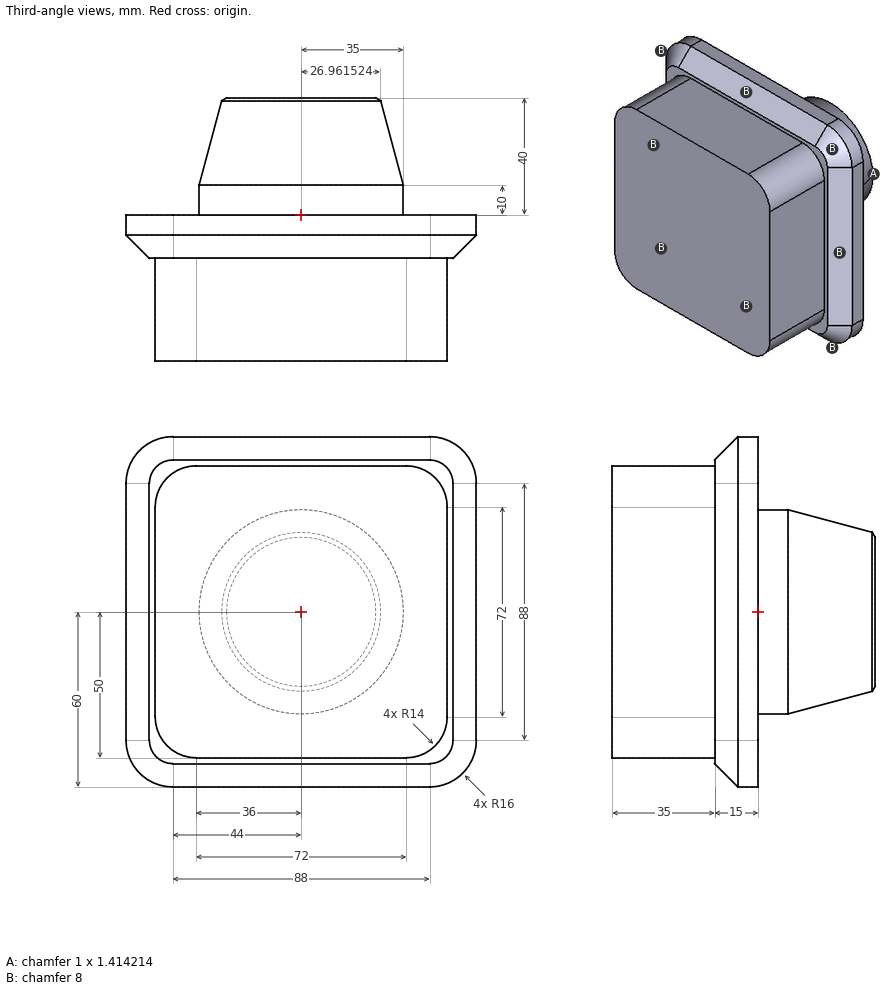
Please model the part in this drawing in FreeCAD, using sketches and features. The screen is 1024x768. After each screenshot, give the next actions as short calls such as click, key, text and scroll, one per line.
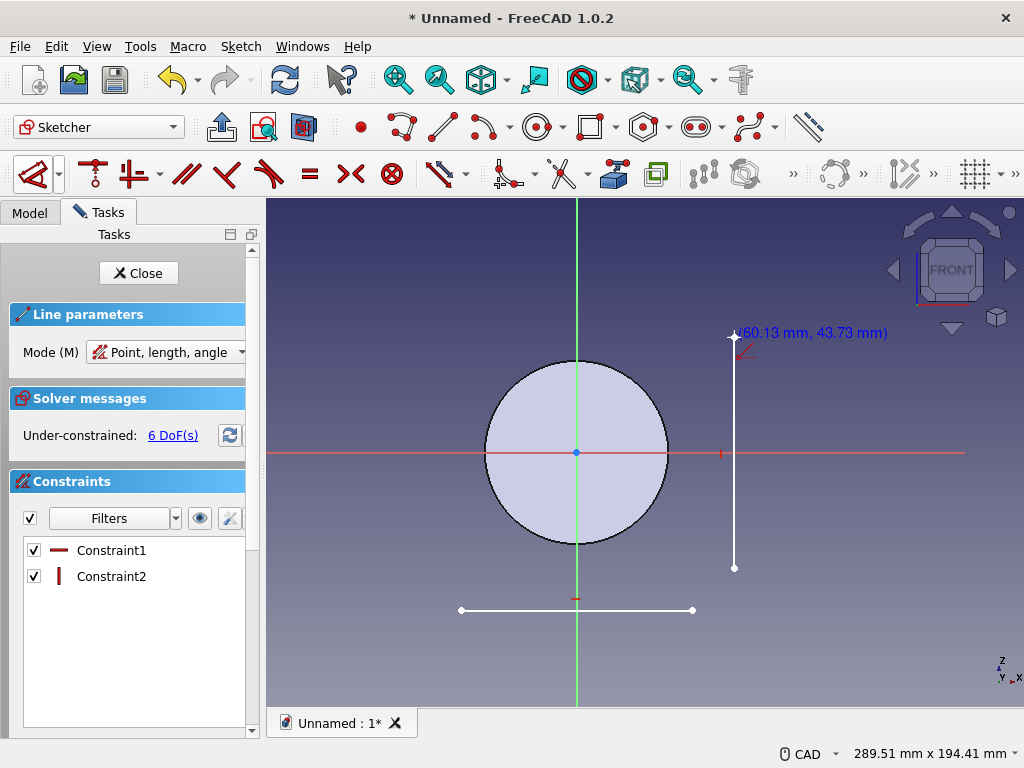
click(692, 295)
click(461, 295)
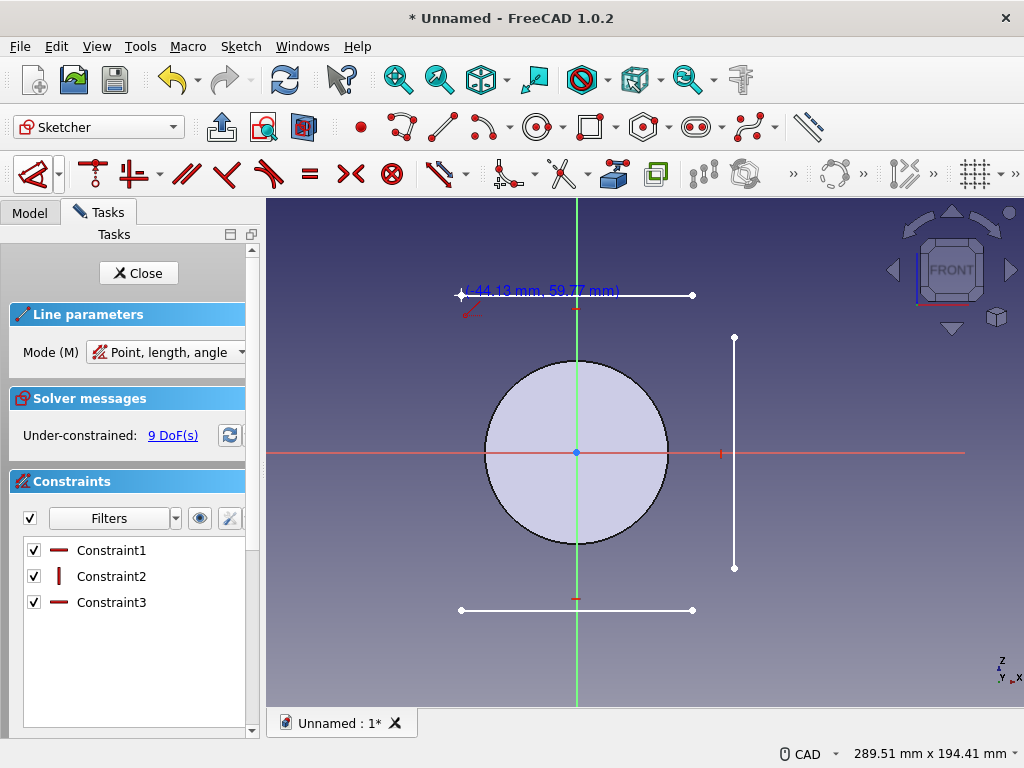
click(419, 337)
click(419, 568)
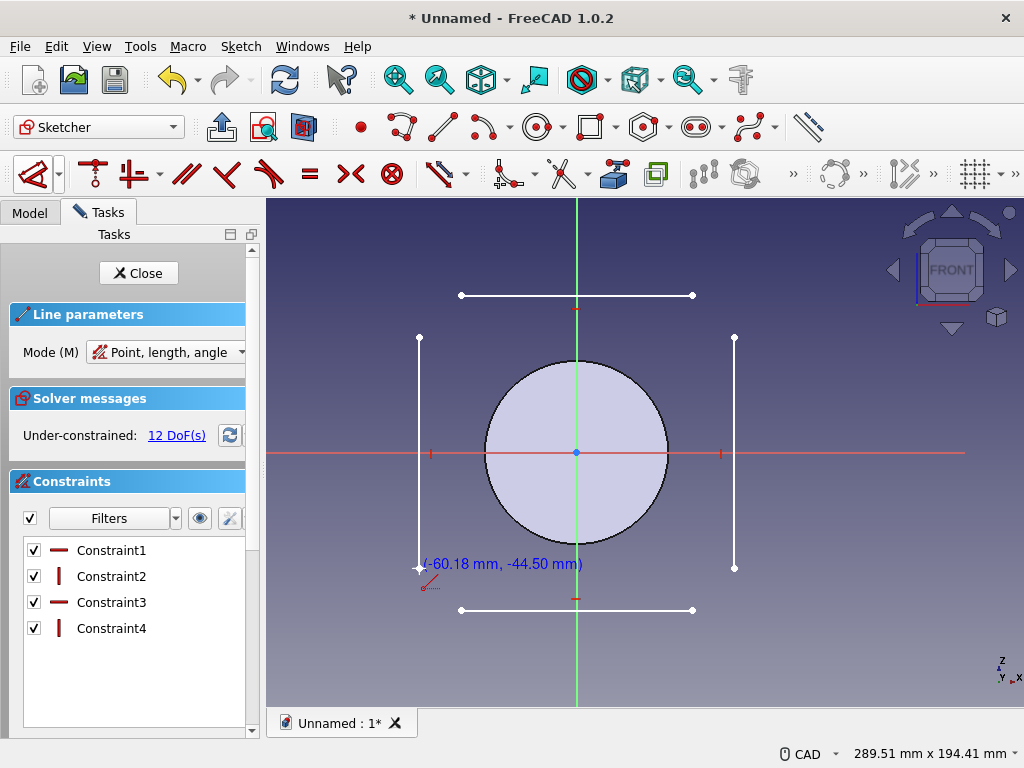
key(g)
key(3)
key(a)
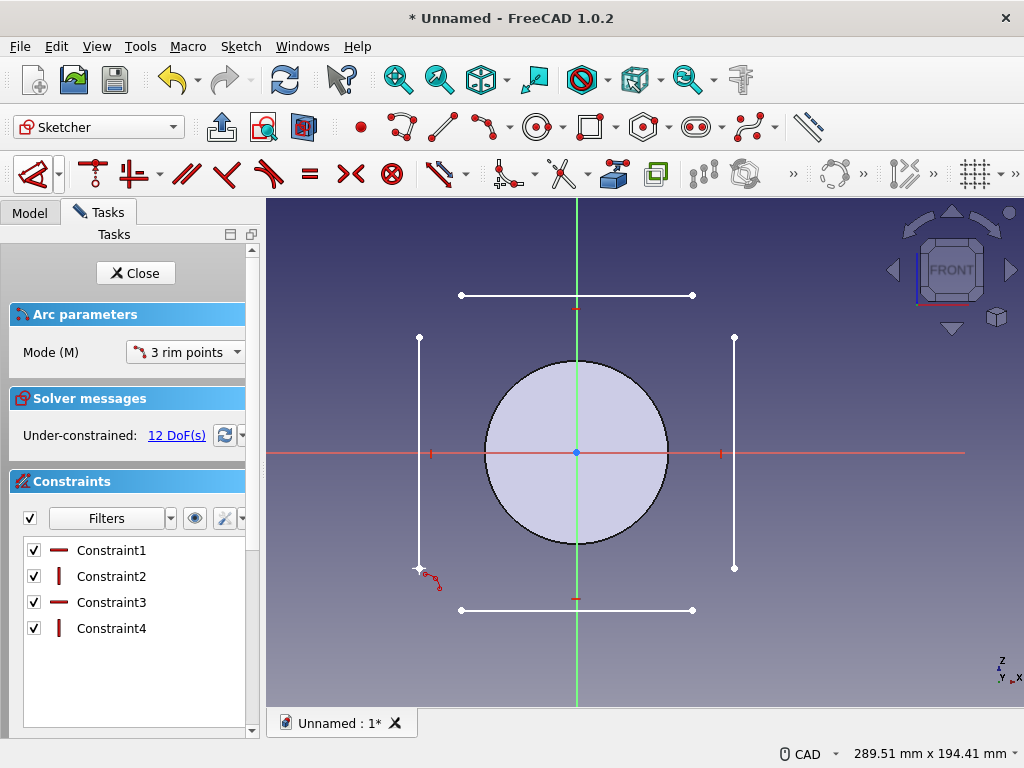
click(692, 611)
click(734, 569)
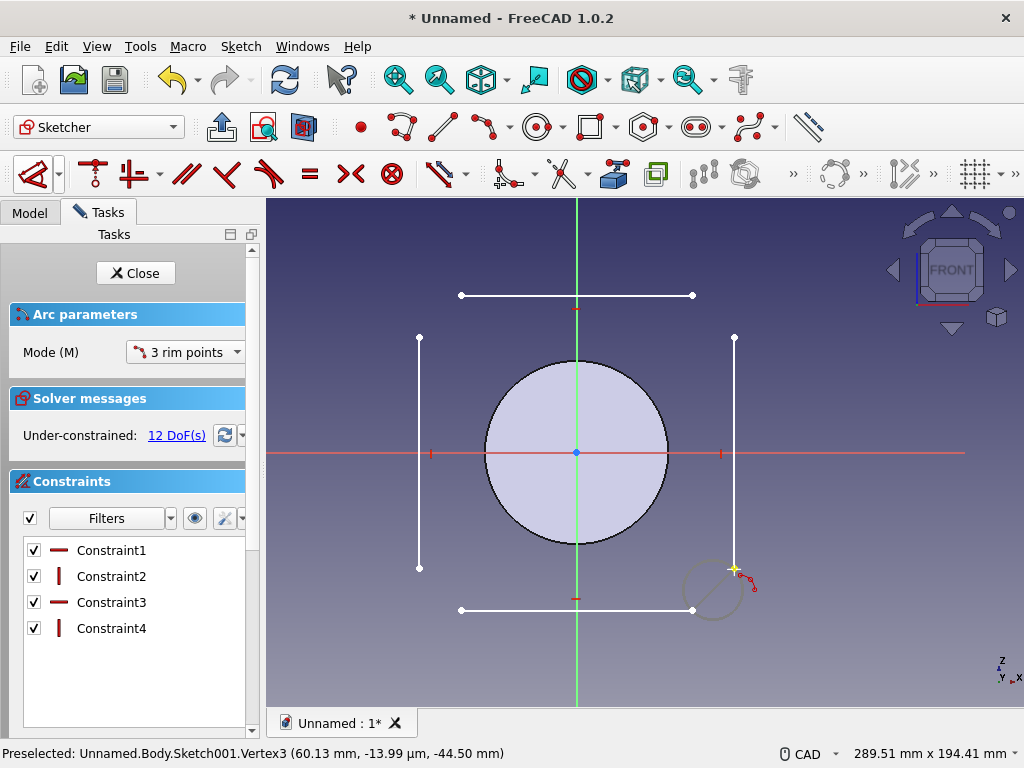
scroll(721, 597, up, 2)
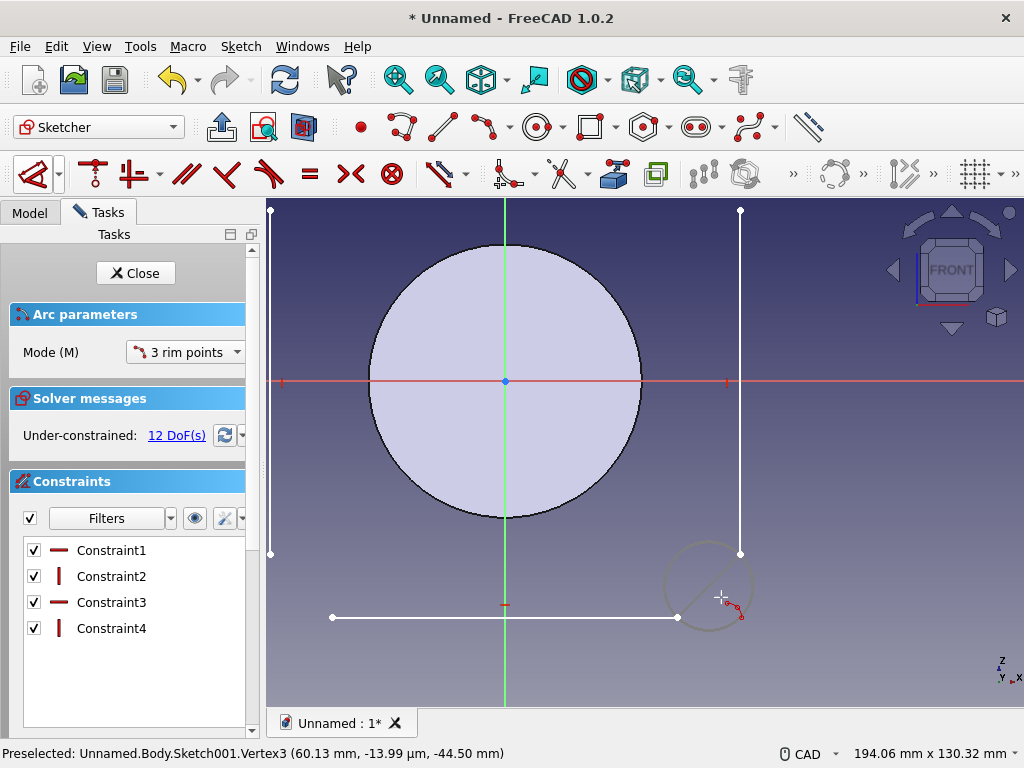
click(721, 597)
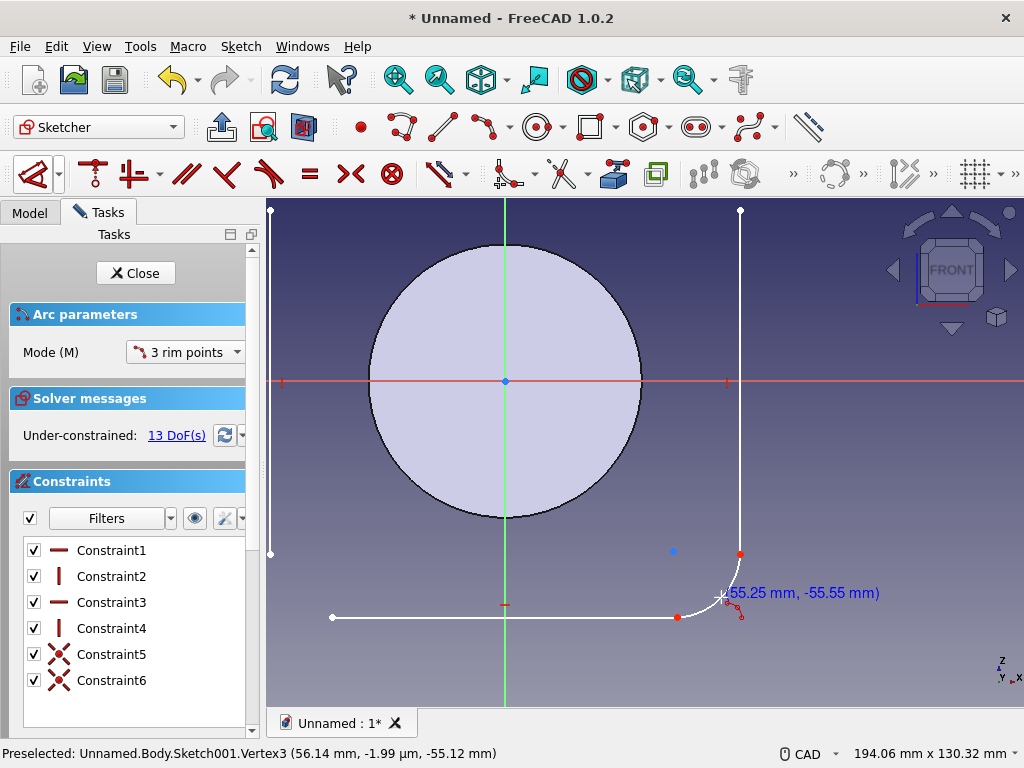
scroll(721, 598, down, 2)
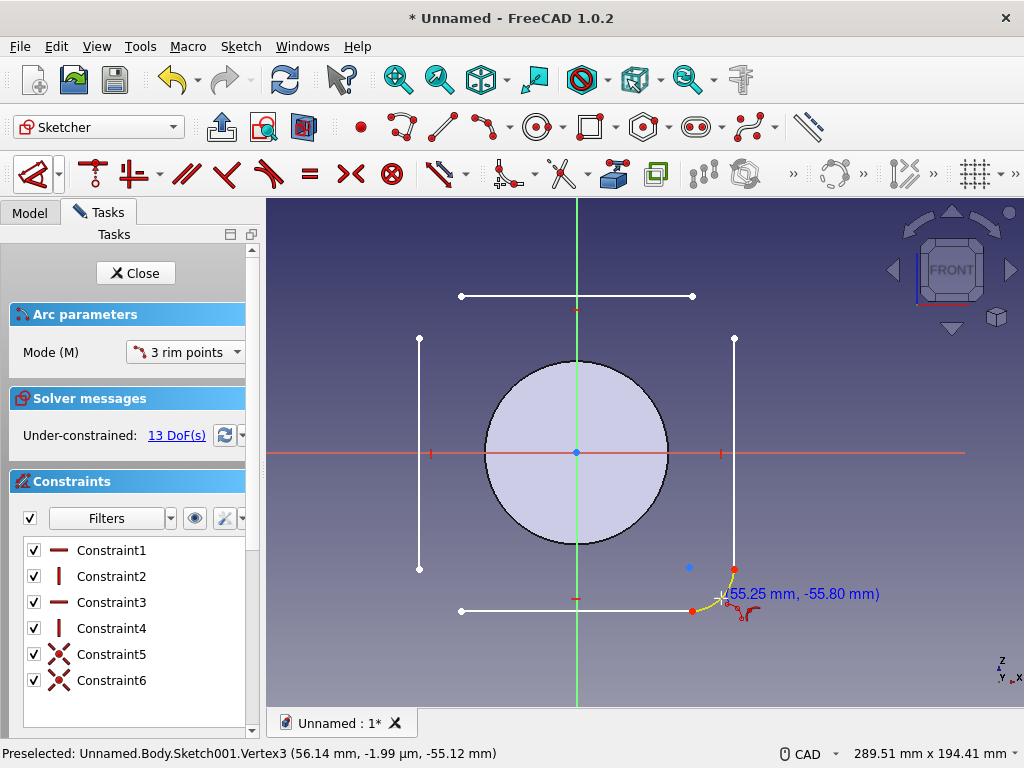
click(734, 338)
click(692, 296)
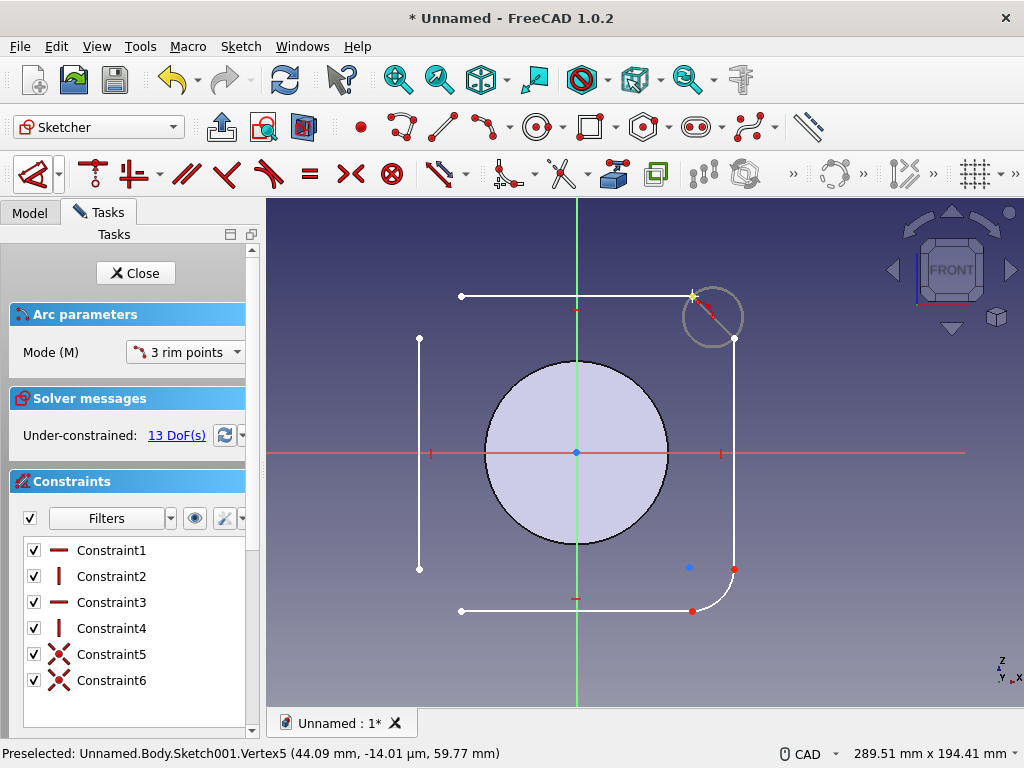
scroll(721, 308, up, 2)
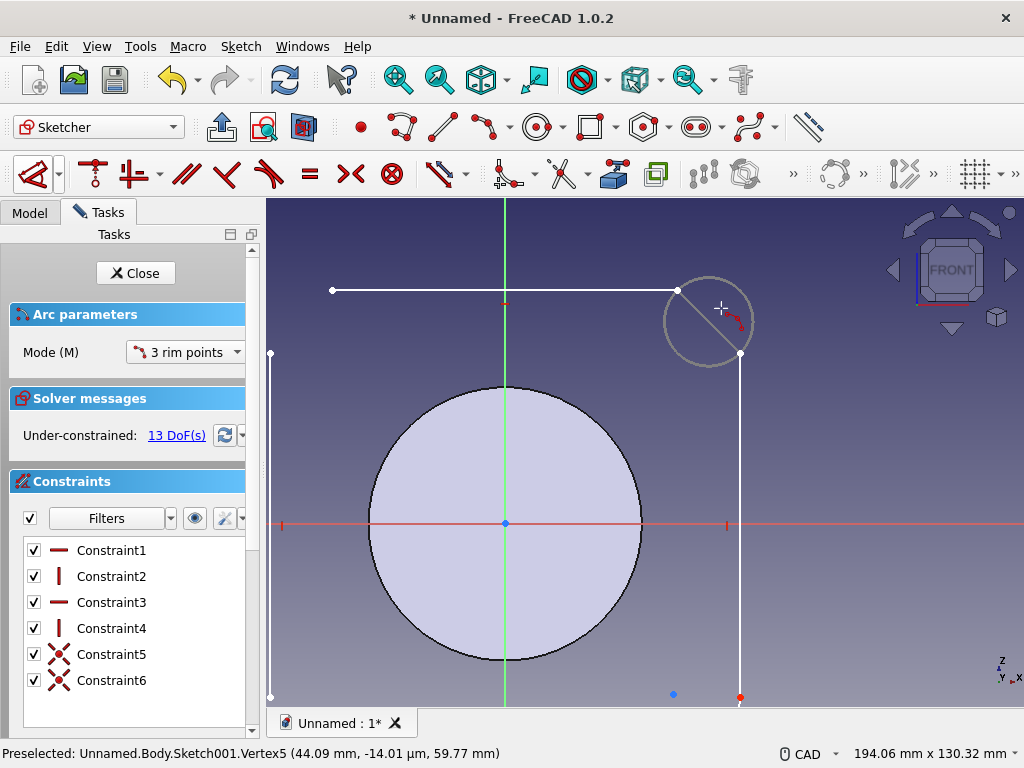
click(721, 308)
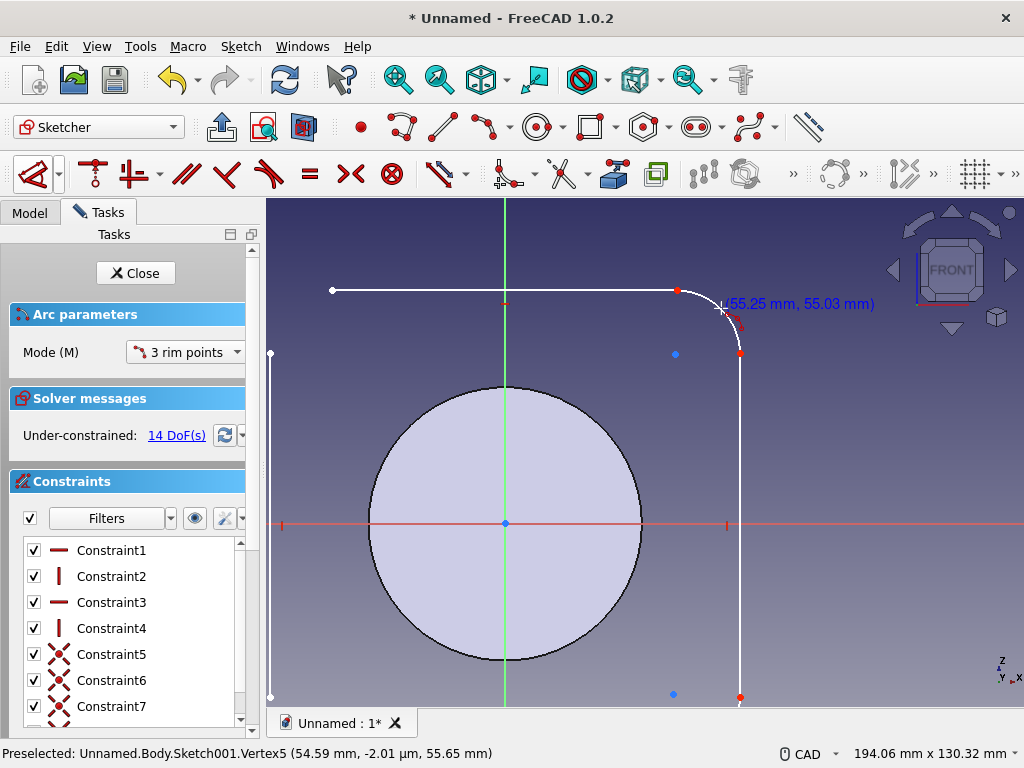
click(333, 290)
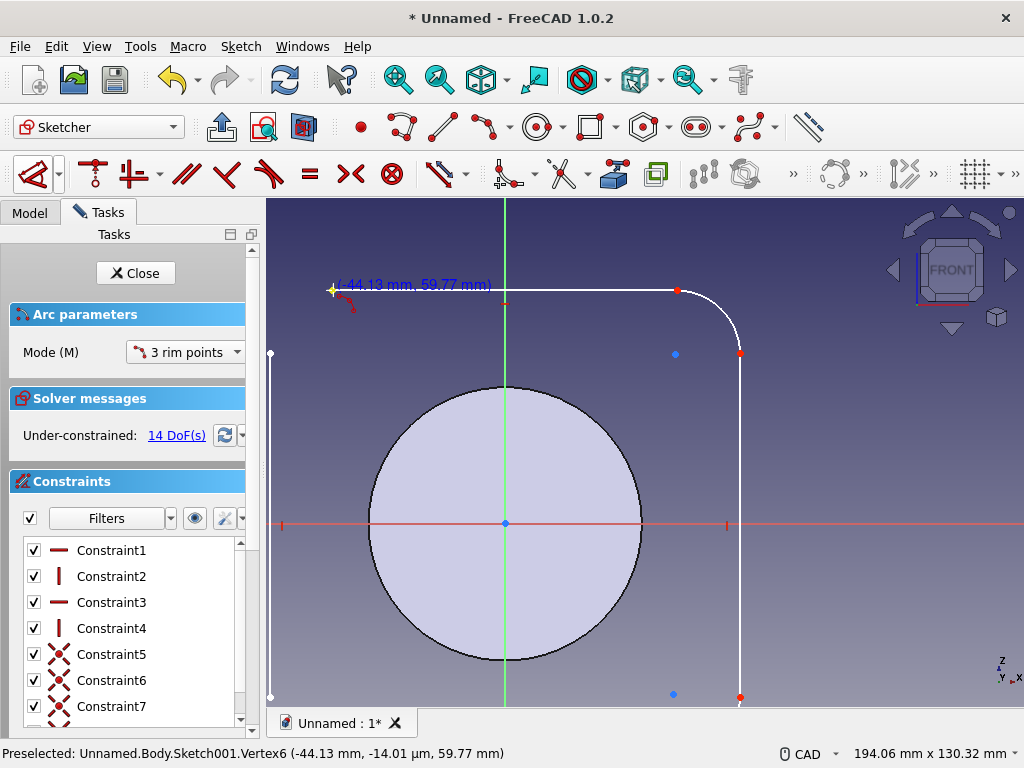
scroll(721, 307, down, 2)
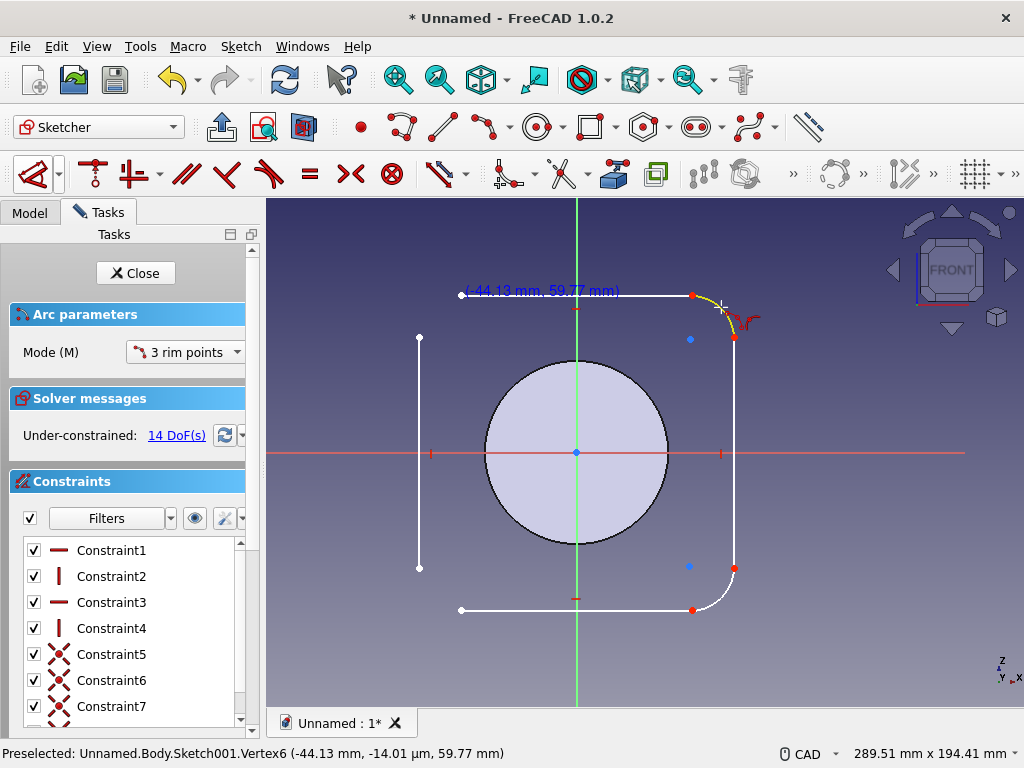
click(419, 338)